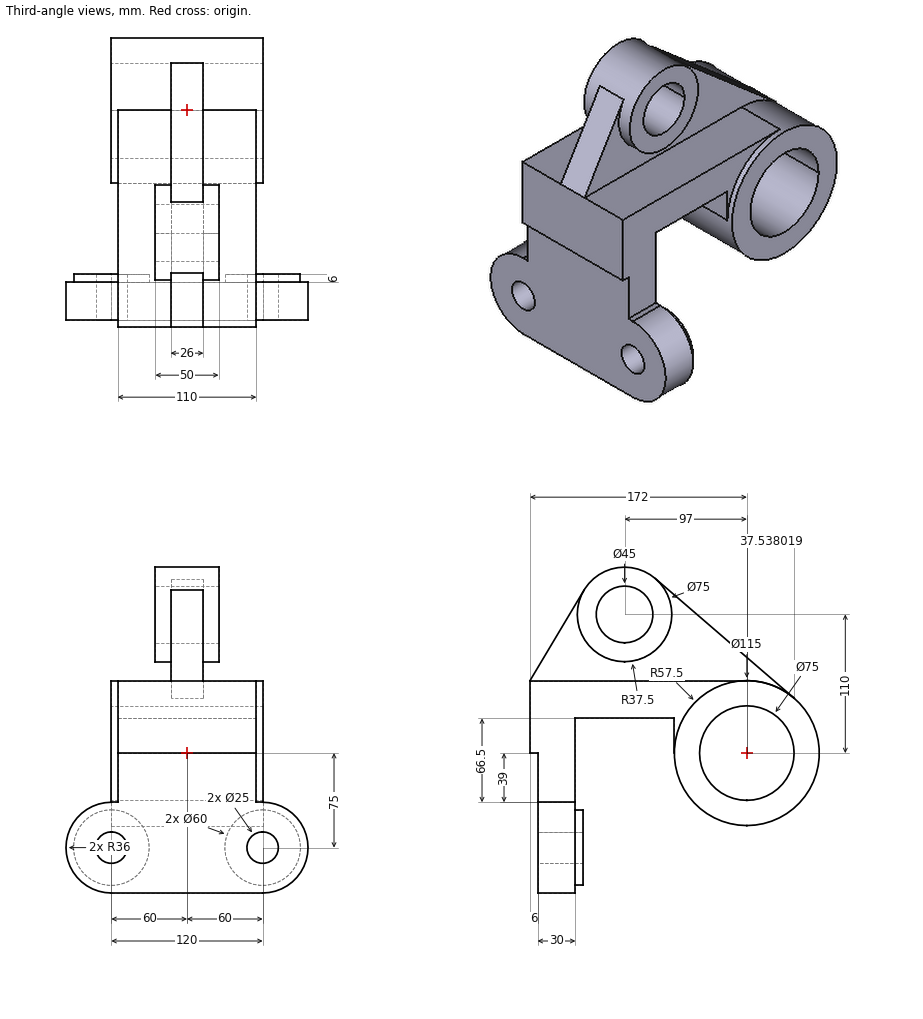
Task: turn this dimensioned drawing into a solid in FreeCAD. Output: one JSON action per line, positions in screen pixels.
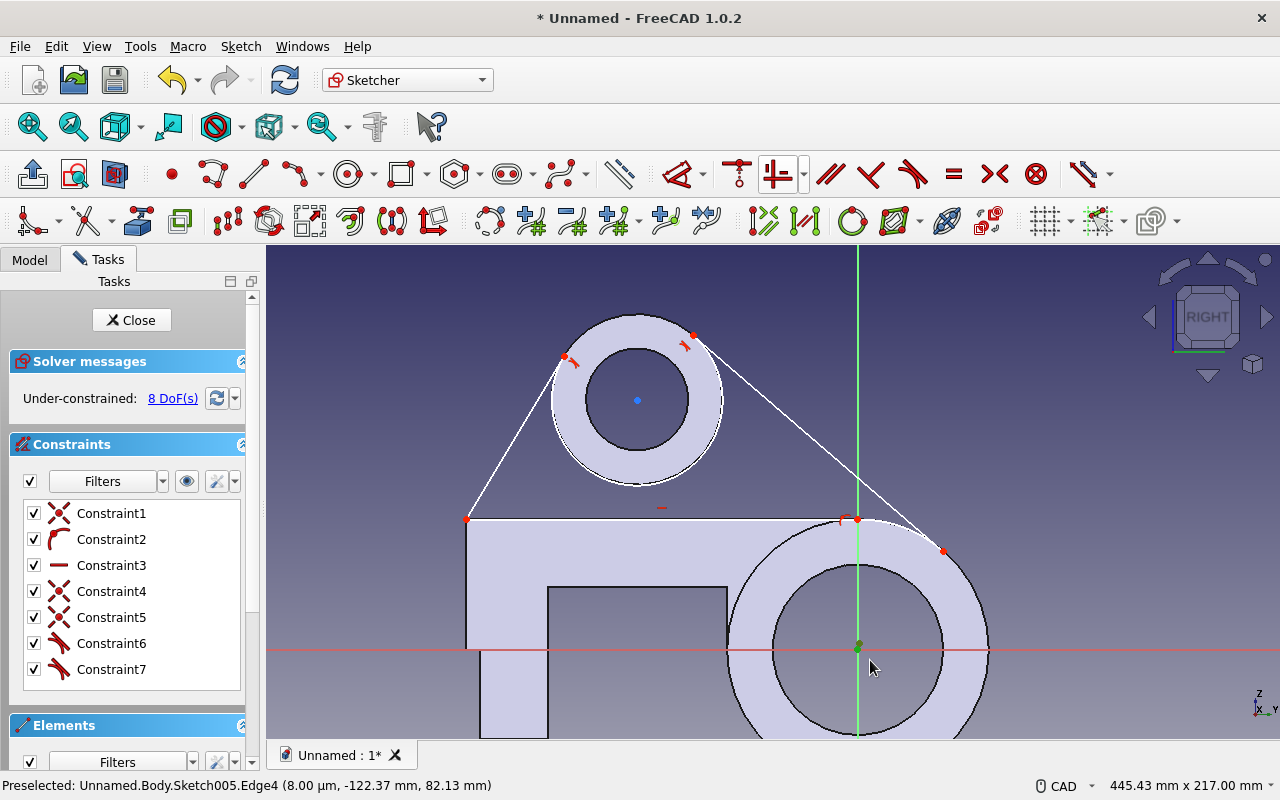
{"action": "left_click", "coordinate": [737, 174]}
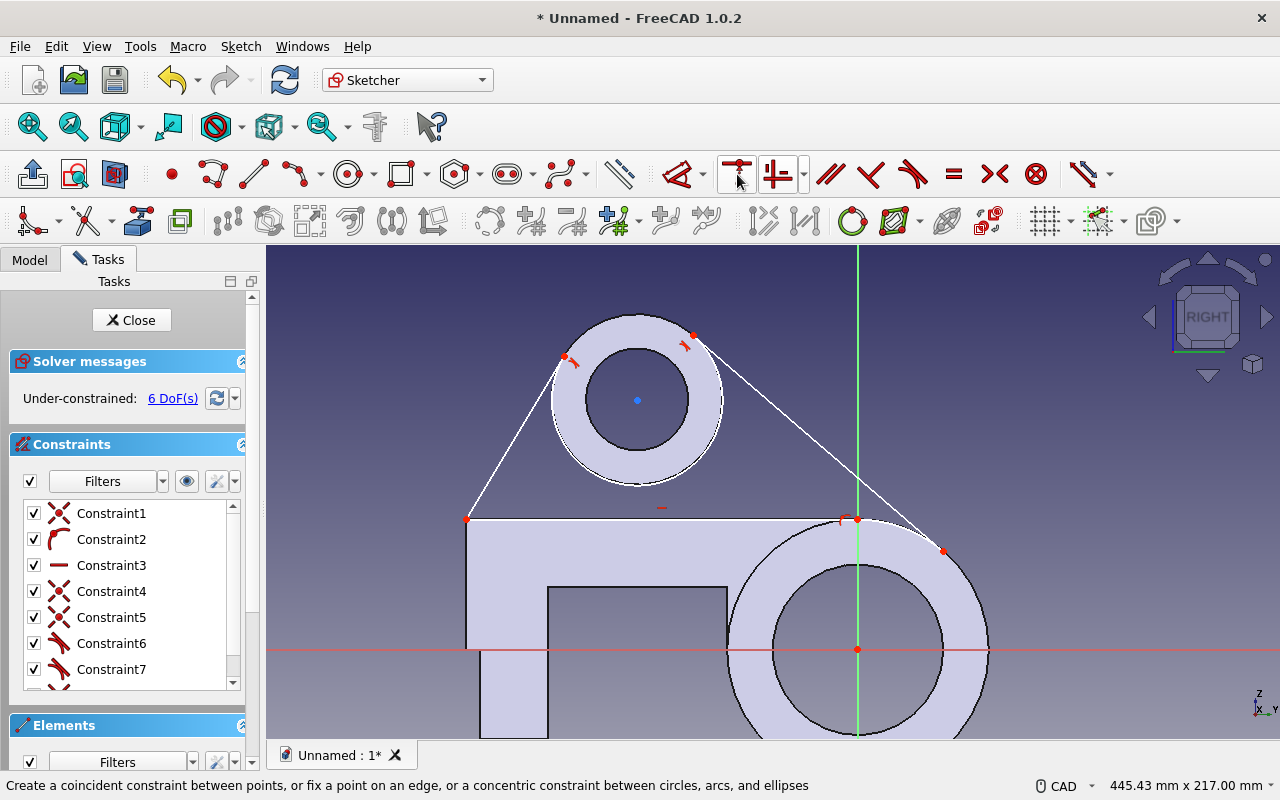
{"action": "key", "text": "d"}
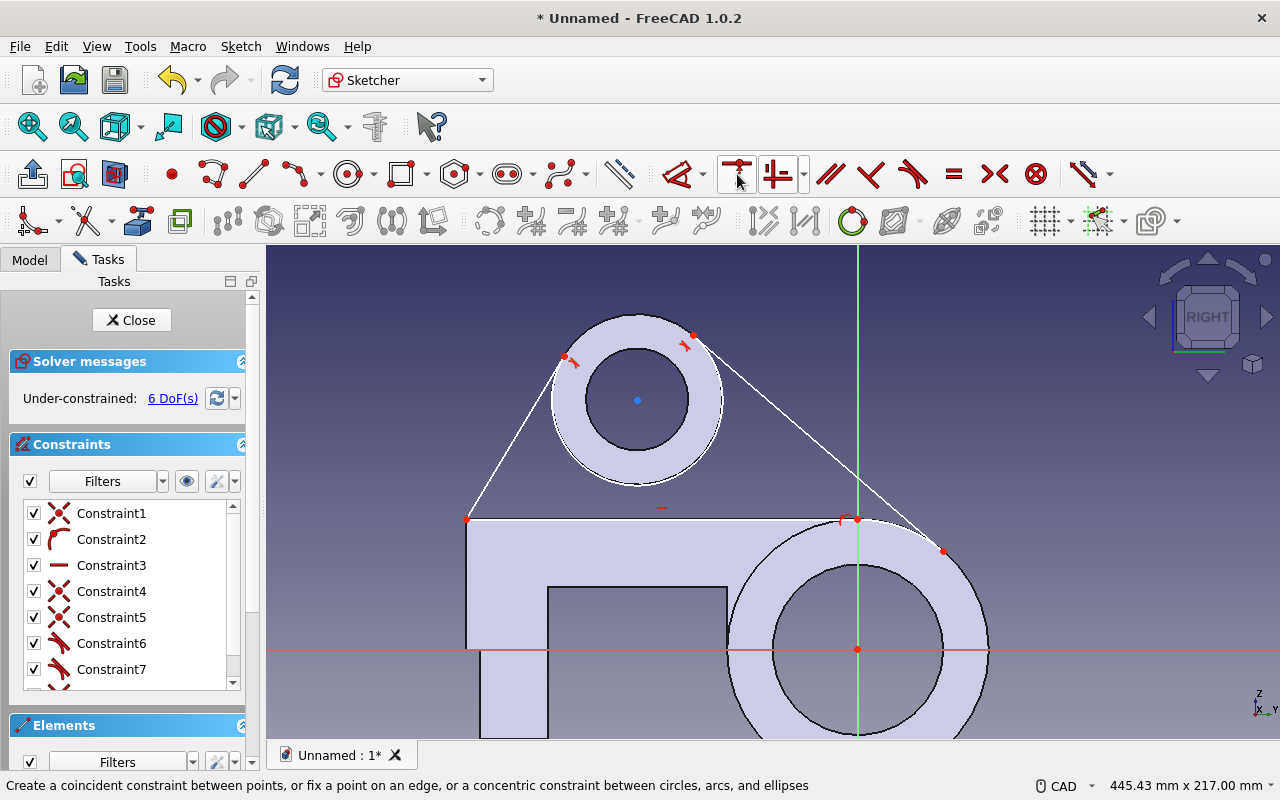
{"action": "left_click", "coordinate": [579, 463]}
{"action": "left_click", "coordinate": [557, 486]}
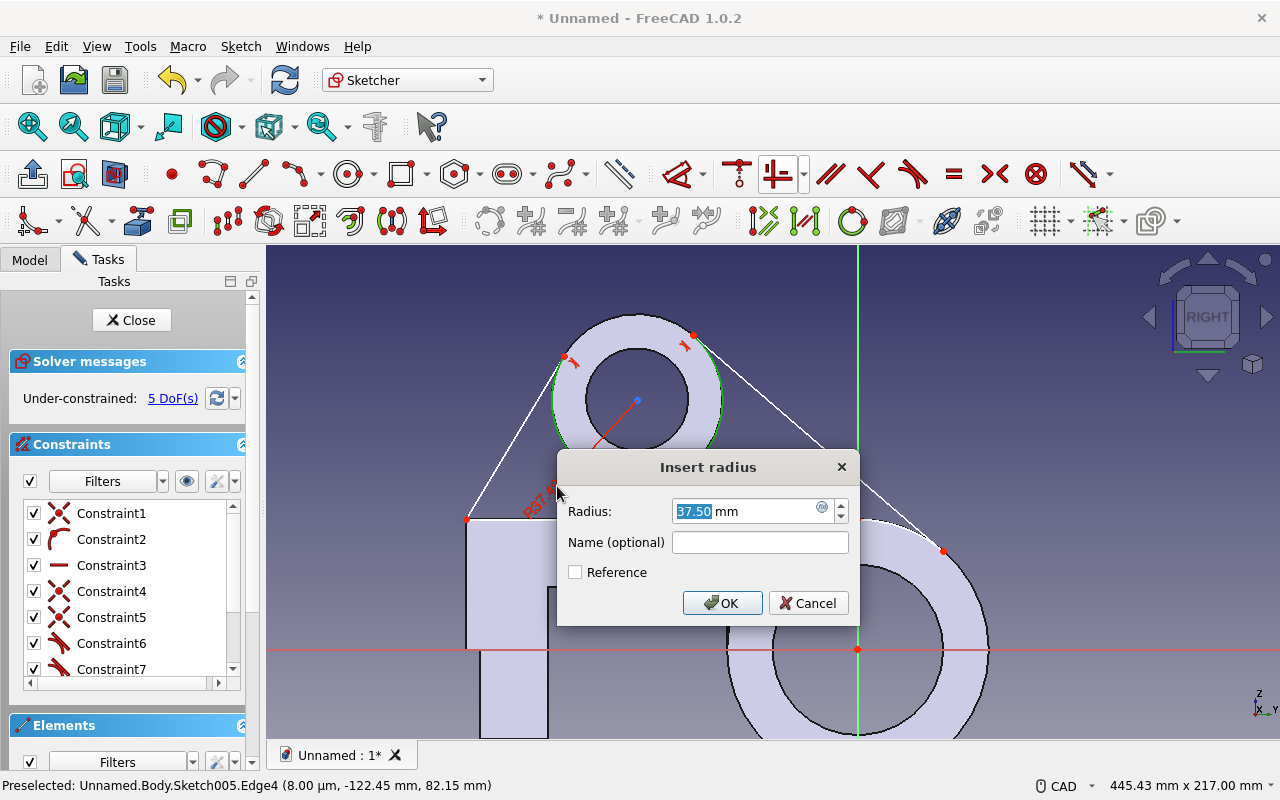
{"action": "type", "text": "37.5"}
{"action": "key", "text": "Return"}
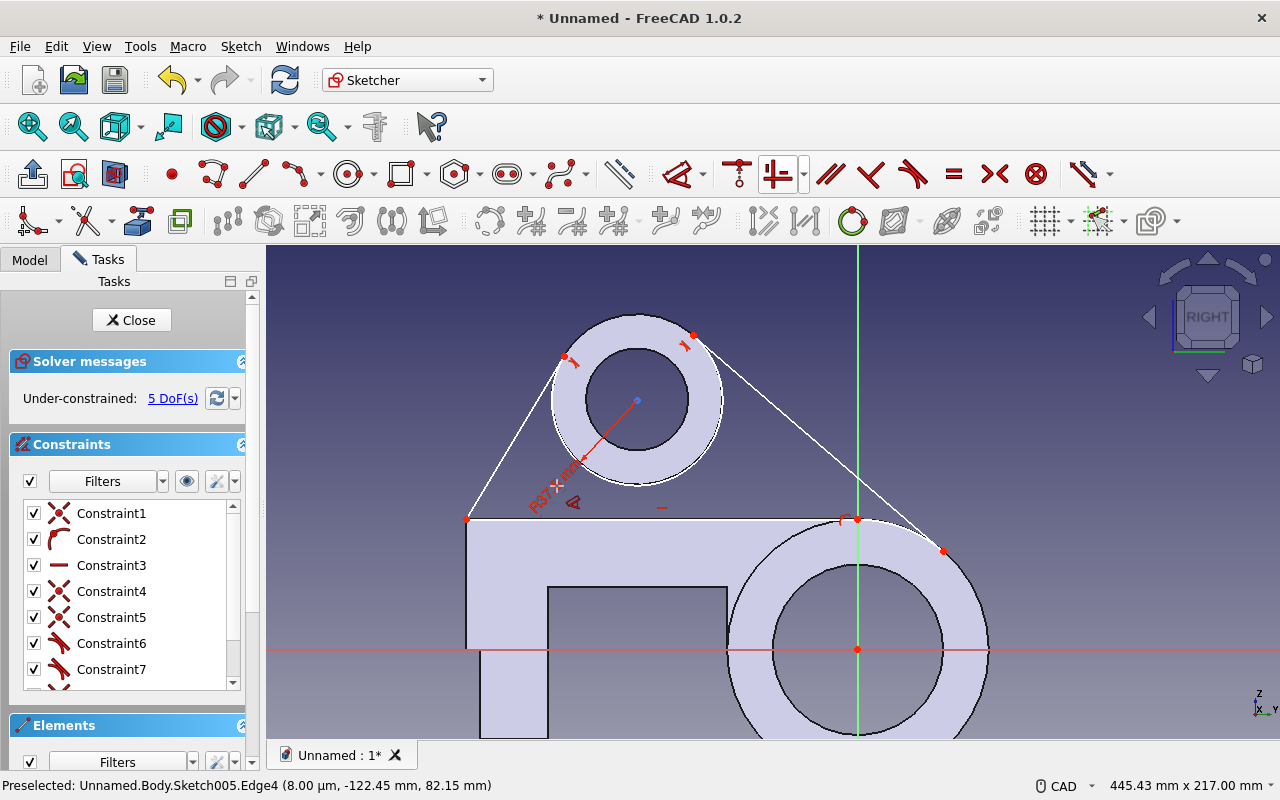
{"action": "left_click", "coordinate": [886, 523]}
{"action": "left_click", "coordinate": [964, 528]}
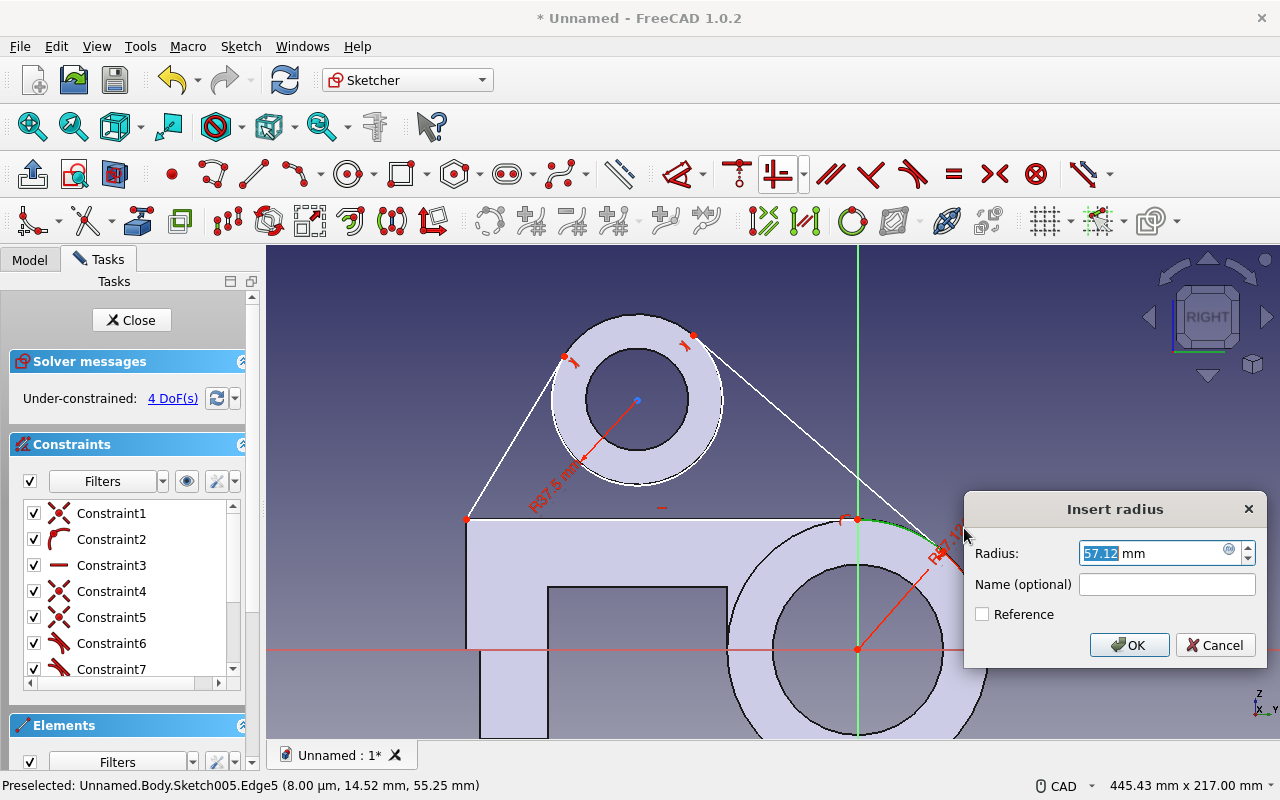
{"action": "type", "text": "57.5"}
{"action": "key", "text": "Return"}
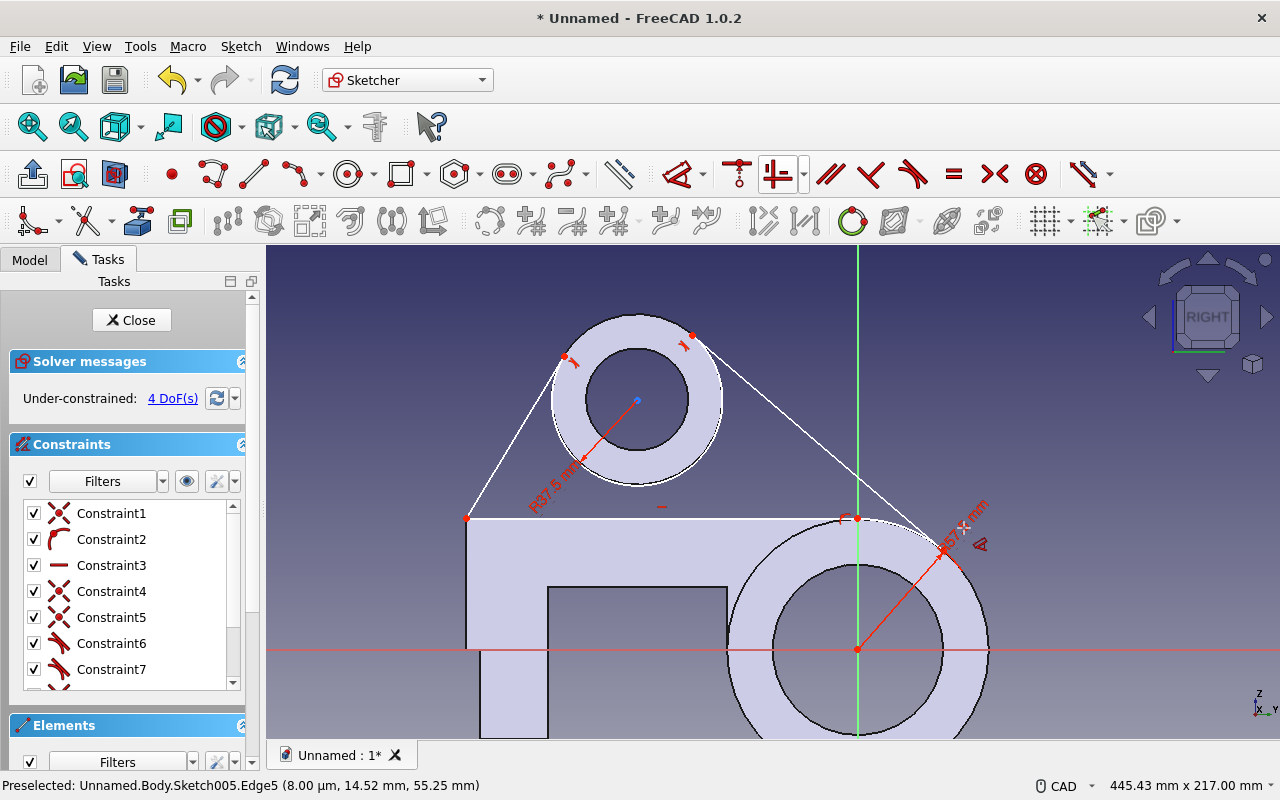
{"action": "left_click", "coordinate": [584, 519]}
{"action": "left_click", "coordinate": [662, 553]}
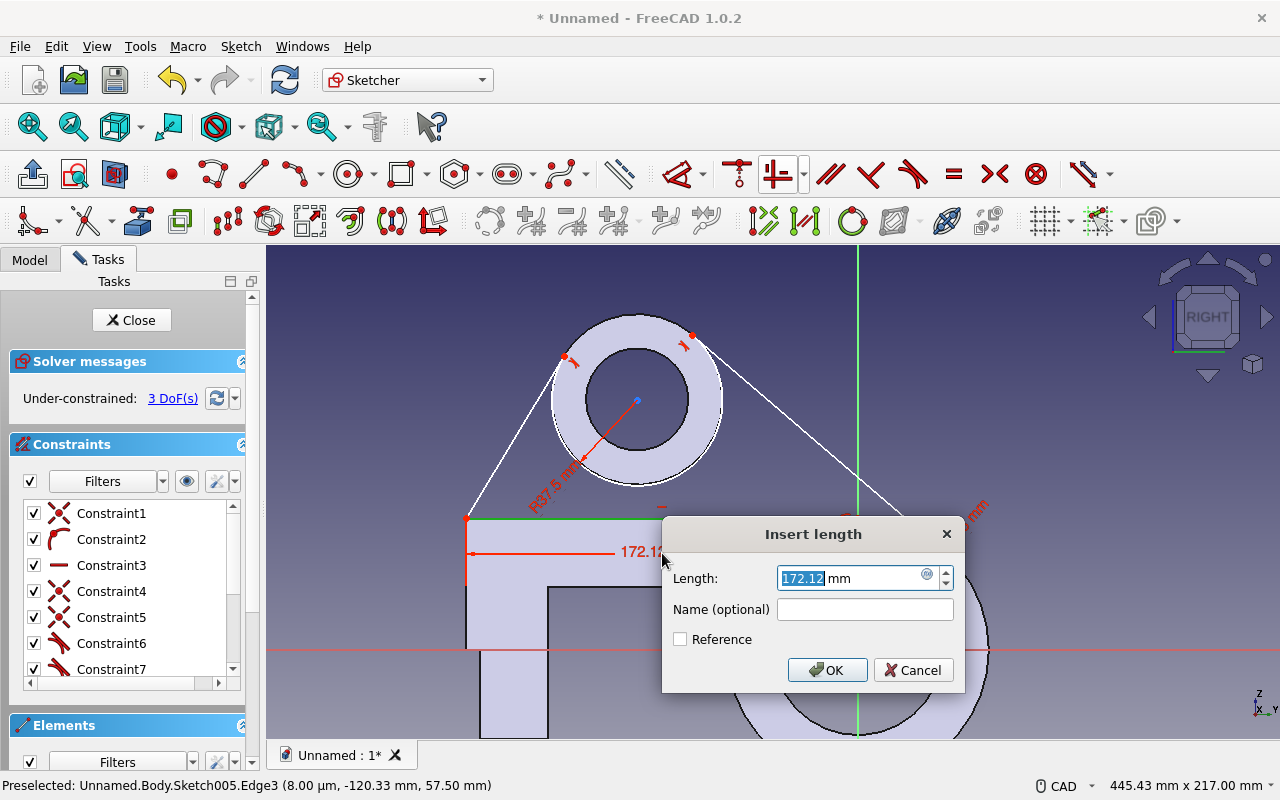
{"action": "type", "text": "172"}
{"action": "key", "text": "Return"}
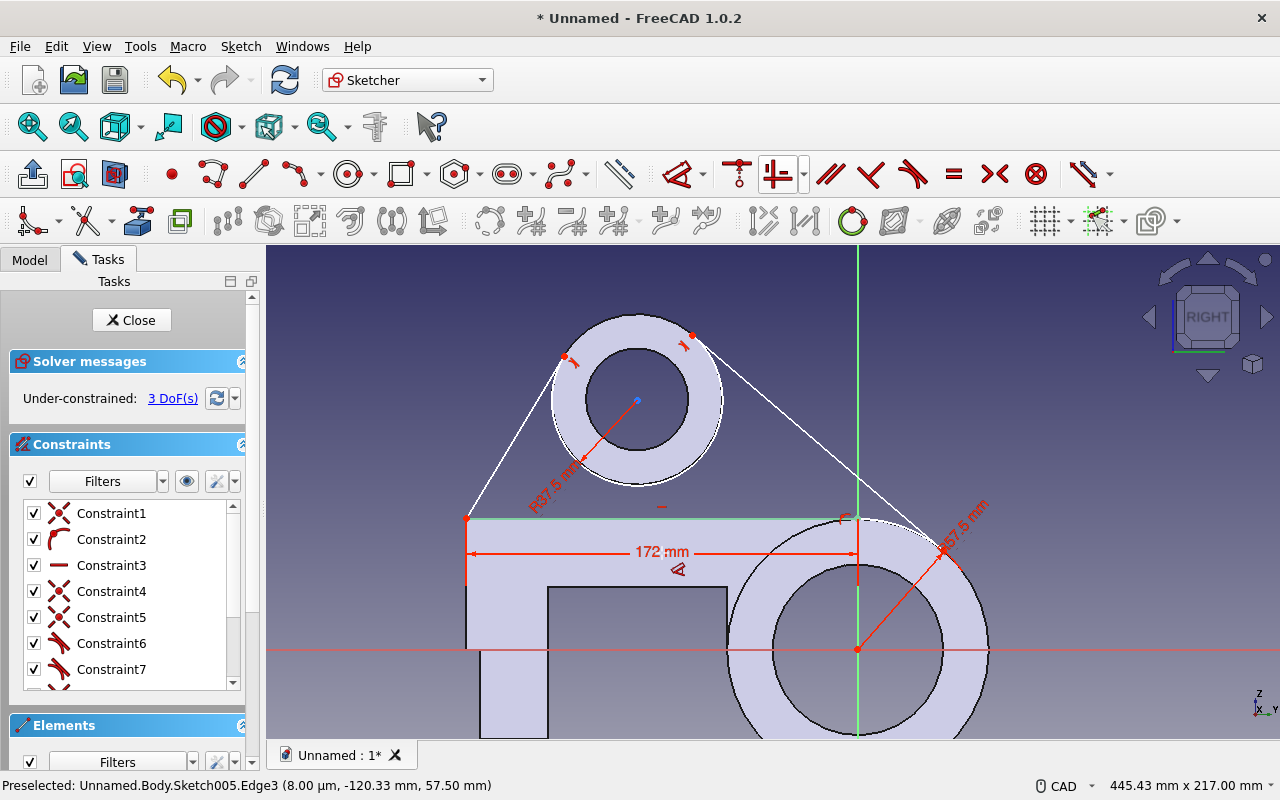
{"action": "left_click", "coordinate": [637, 400]}
{"action": "left_click", "coordinate": [748, 684]}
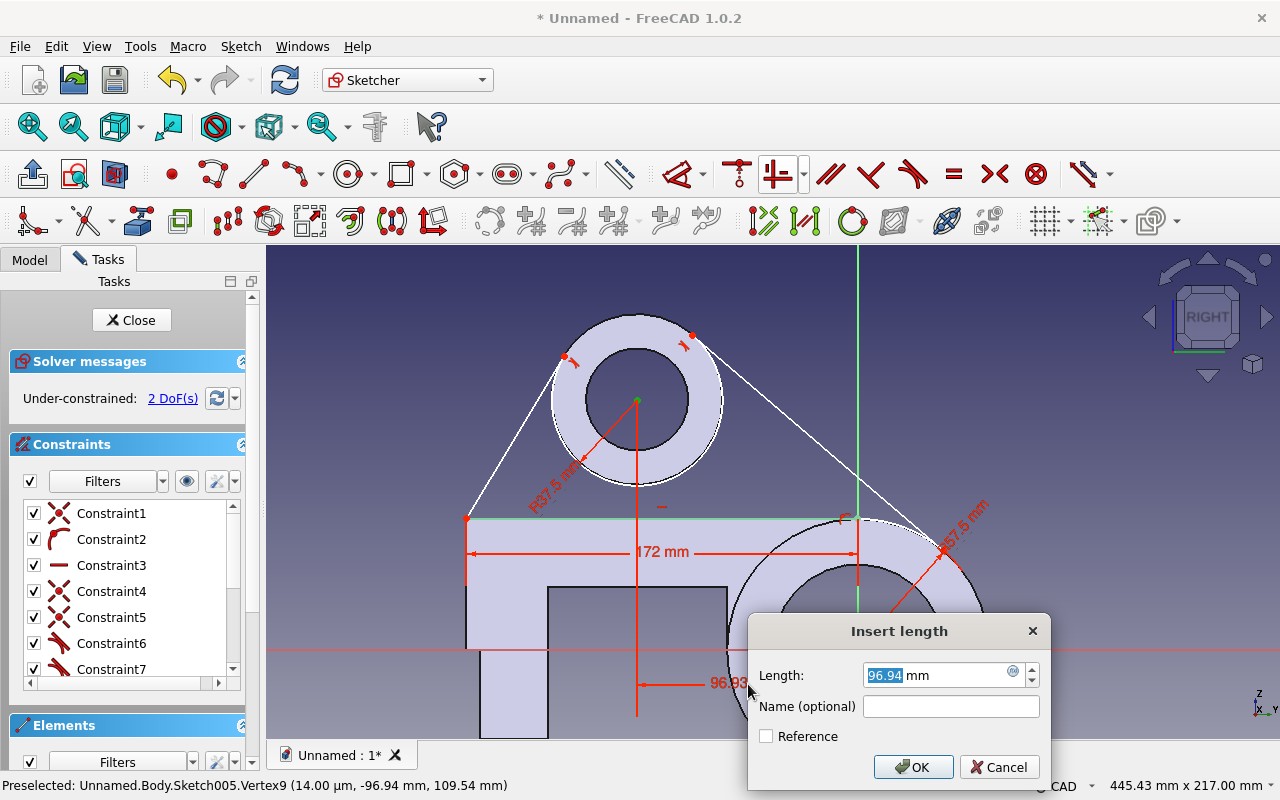
{"action": "type", "text": "97"}
{"action": "key", "text": "Return"}